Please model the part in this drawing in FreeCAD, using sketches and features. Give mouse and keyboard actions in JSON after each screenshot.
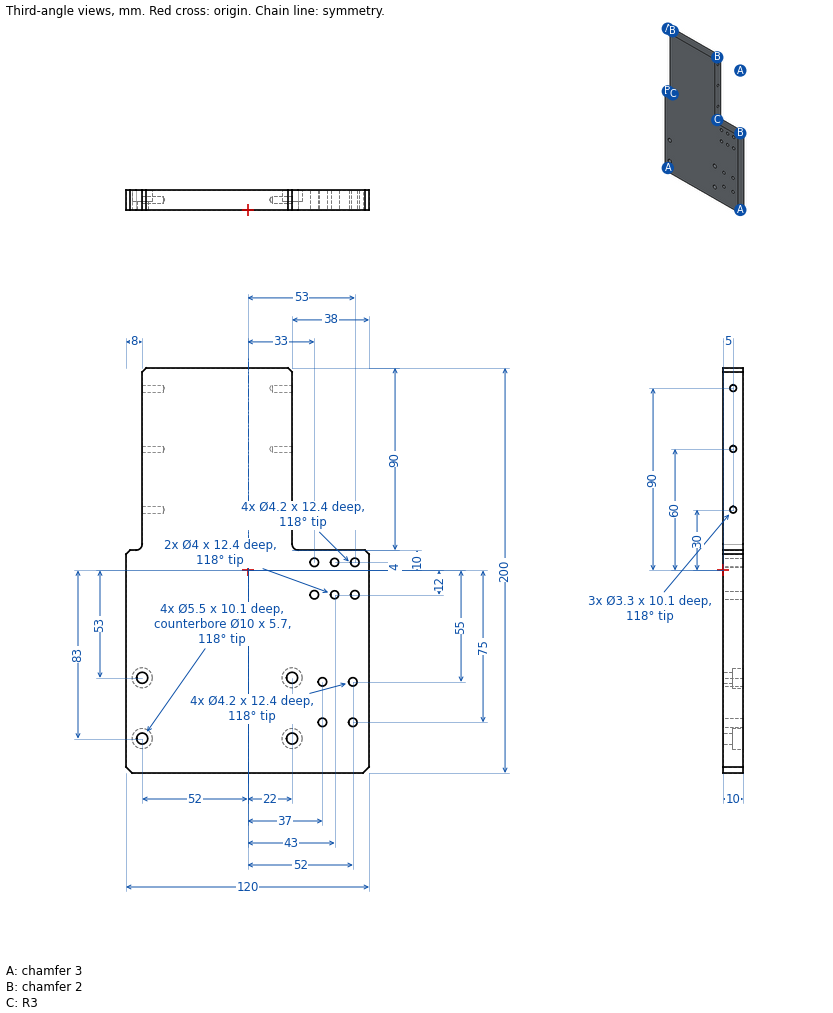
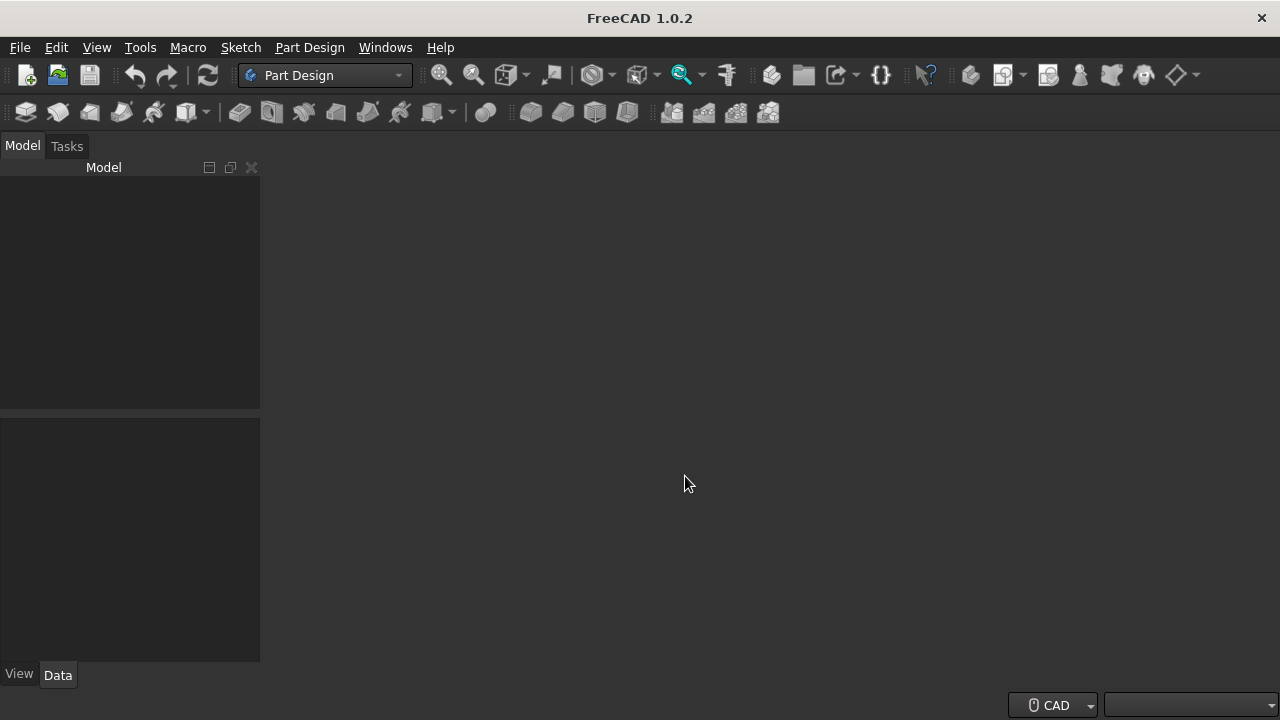
{"action": "left_click", "coordinate": [26, 76]}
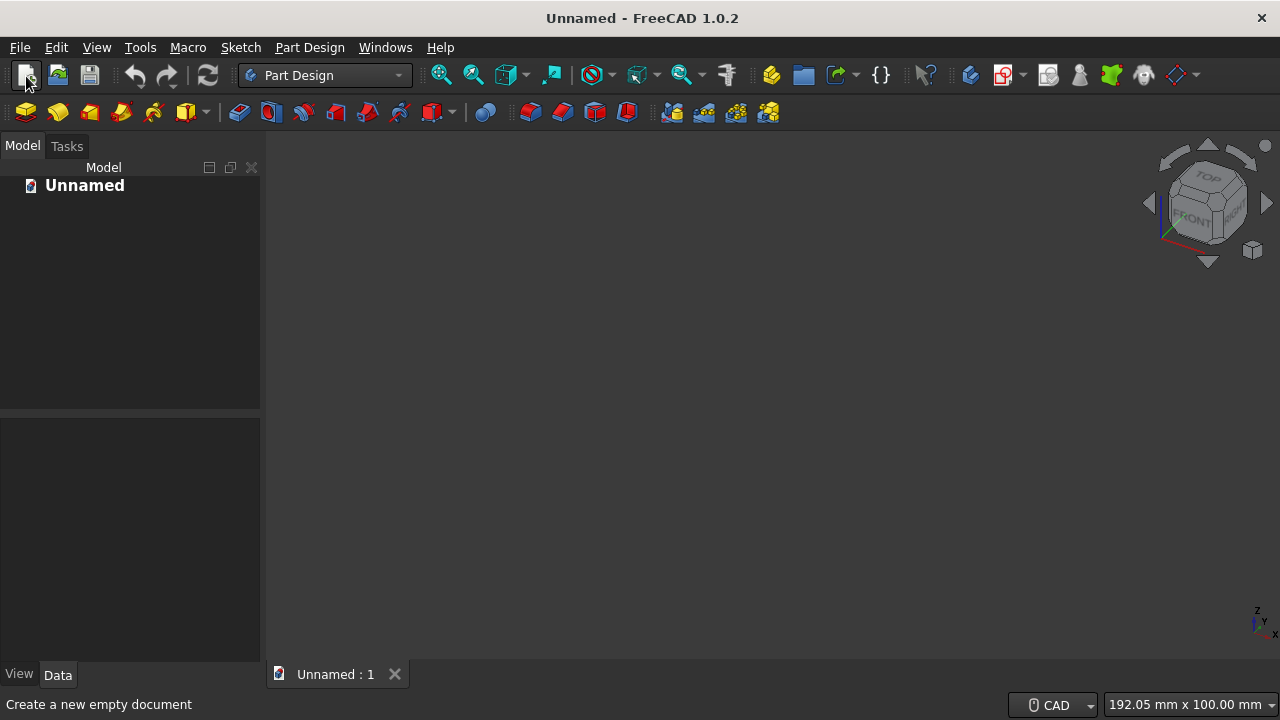
{"action": "left_click", "coordinate": [1004, 76]}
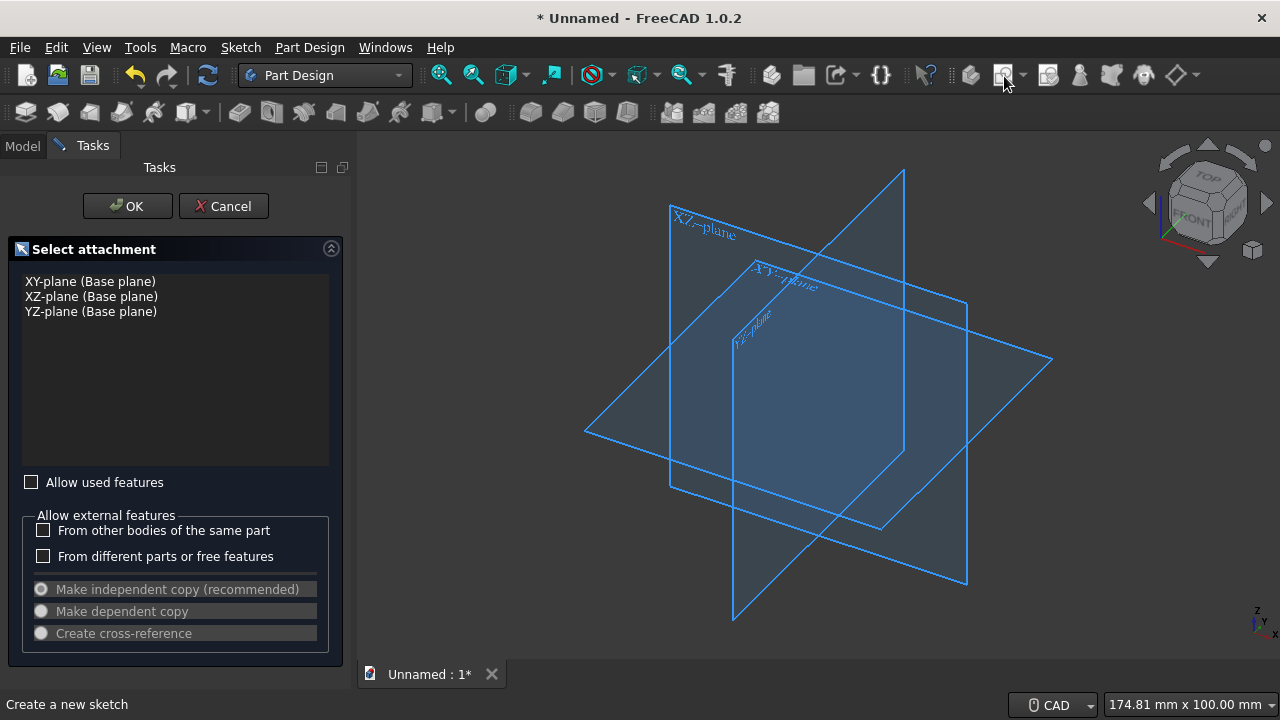
{"action": "left_click", "coordinate": [82, 296]}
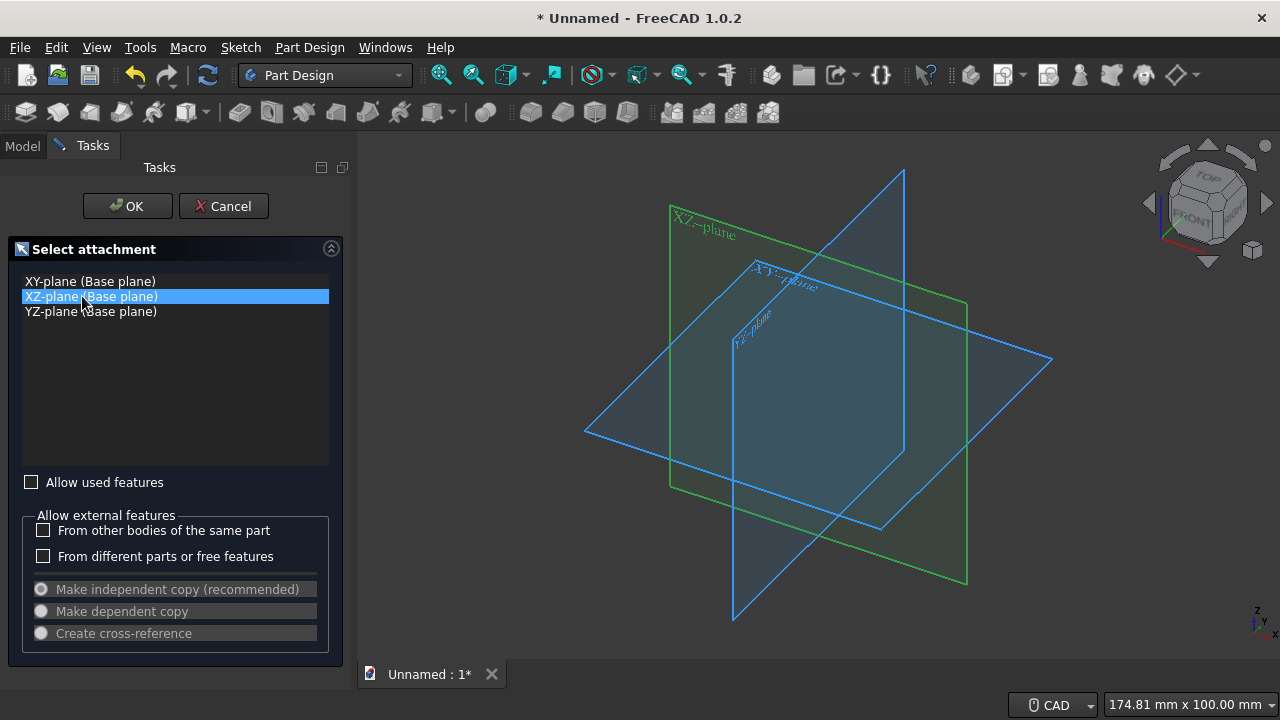
{"action": "left_click", "coordinate": [128, 206]}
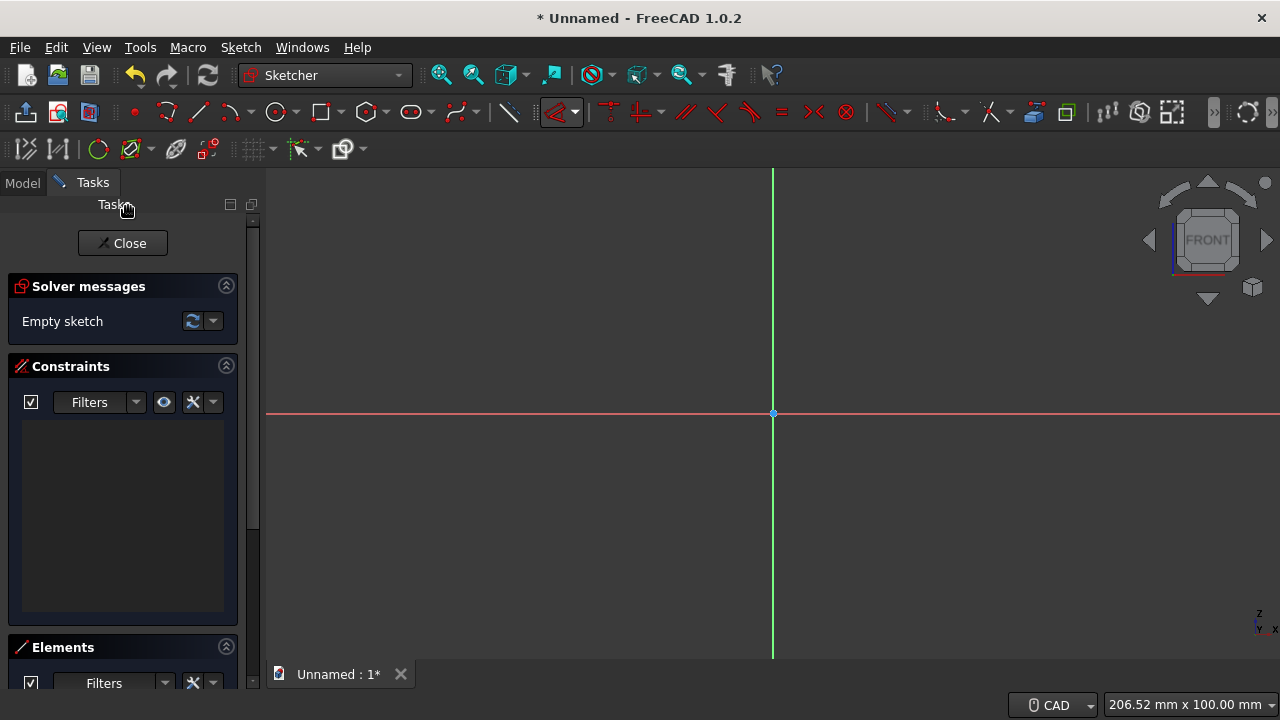
{"action": "scroll", "coordinate": [675, 413], "scroll_direction": "down", "scroll_amount": 6}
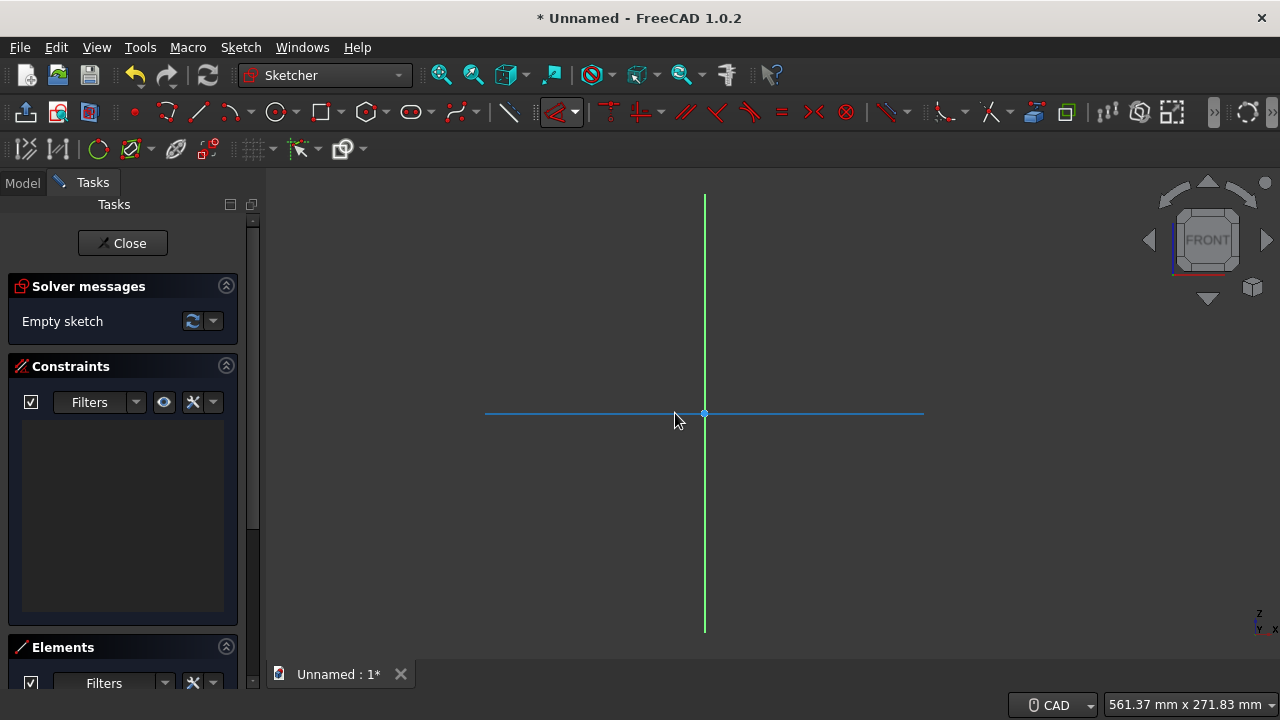
{"action": "key", "text": "g v"}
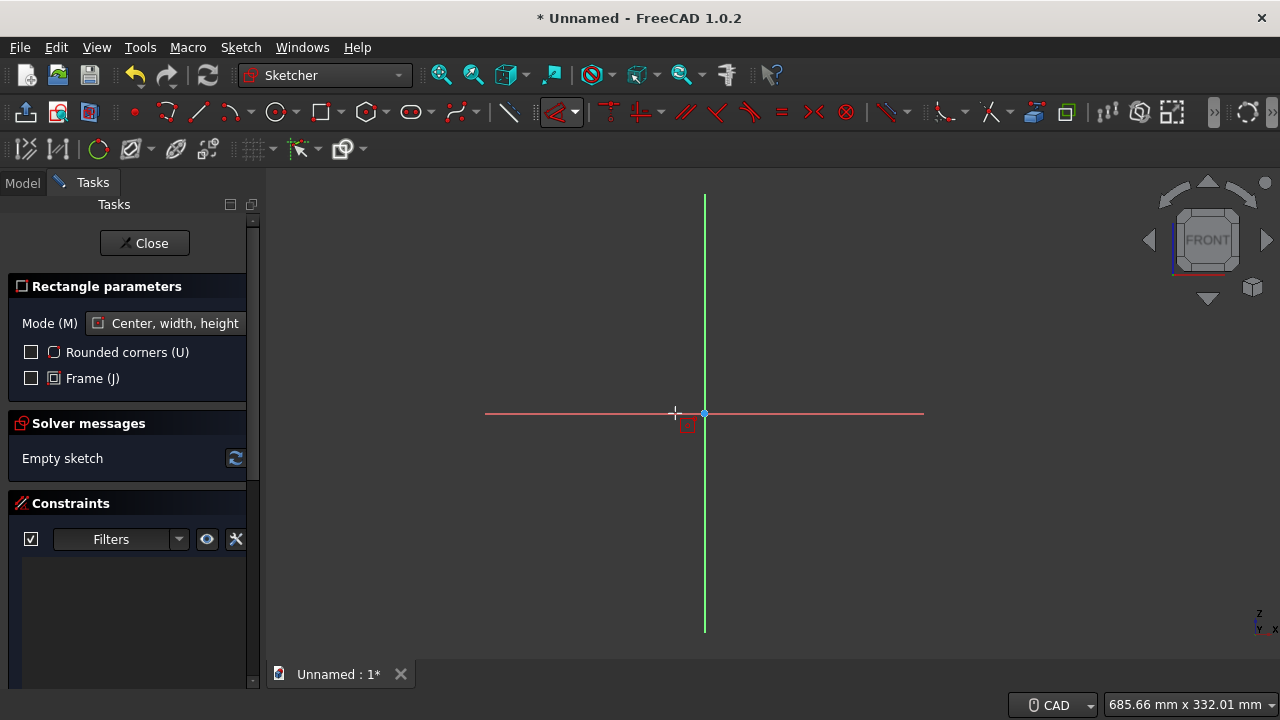
{"action": "left_click", "coordinate": [705, 414]}
{"action": "left_click", "coordinate": [794, 266]}
{"action": "key", "text": "Escape"}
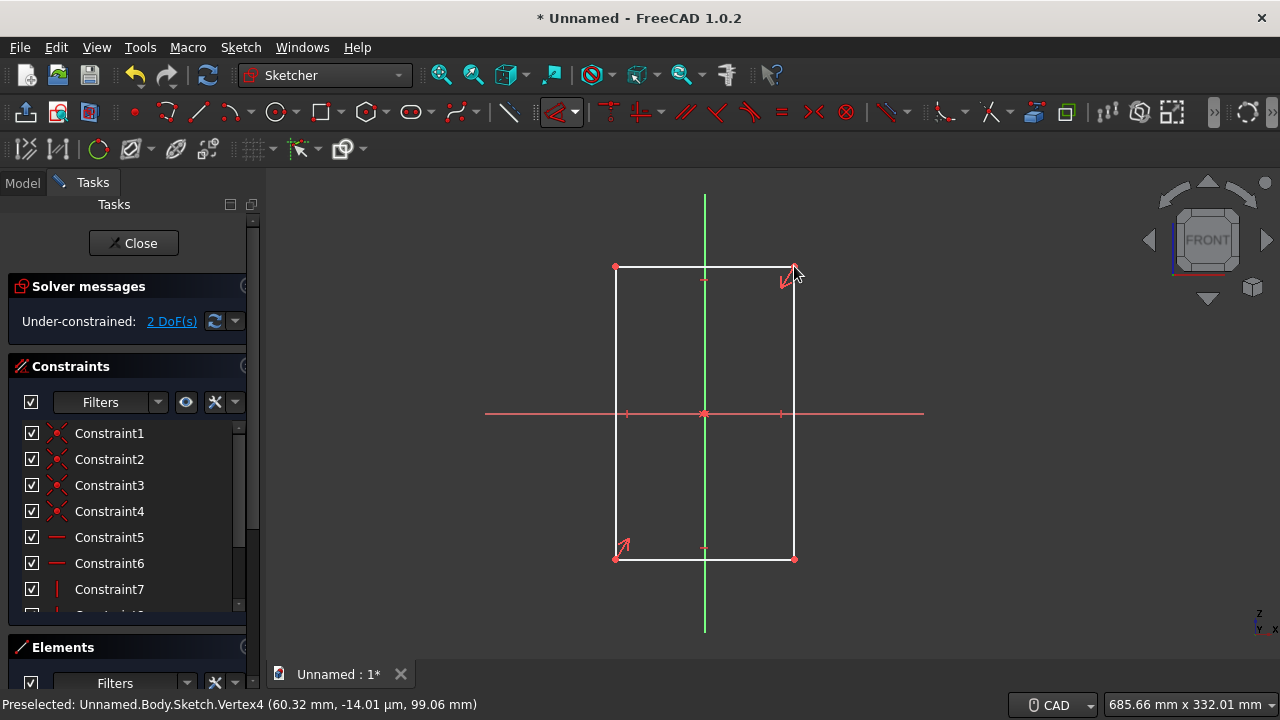
{"action": "left_click", "coordinate": [556, 112]}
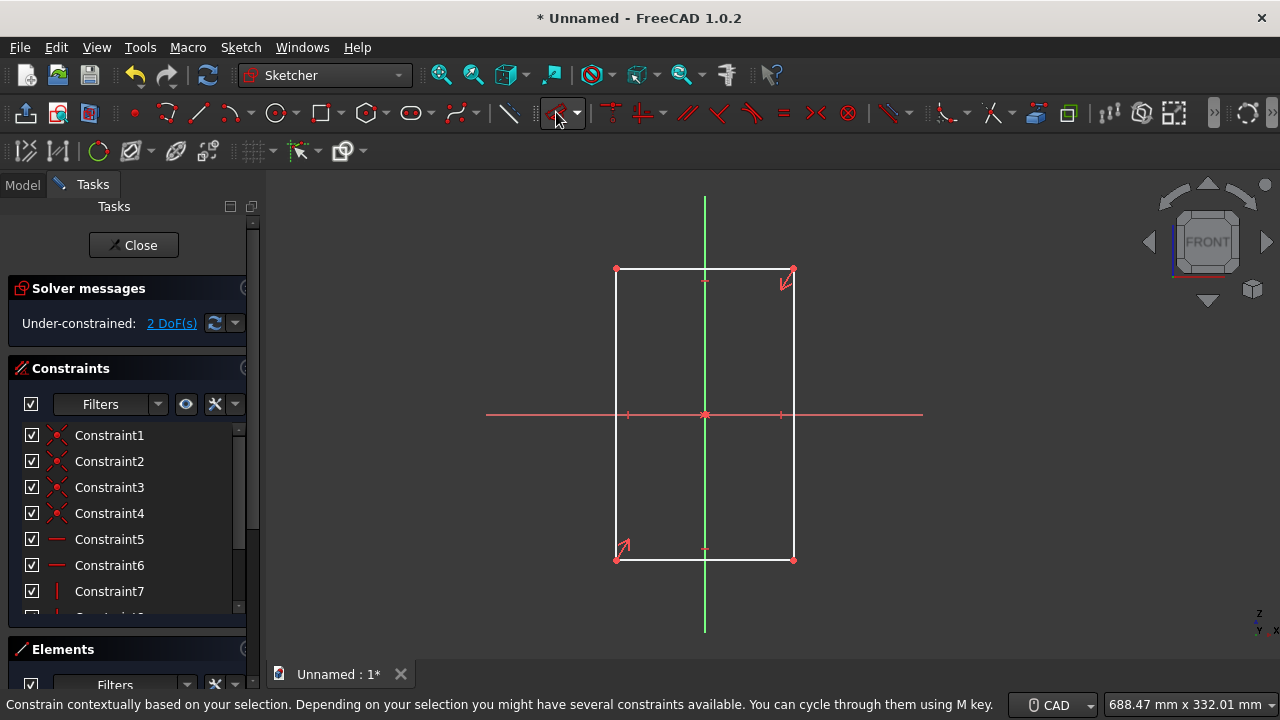
{"action": "left_click", "coordinate": [670, 560]}
{"action": "left_click", "coordinate": [664, 594]}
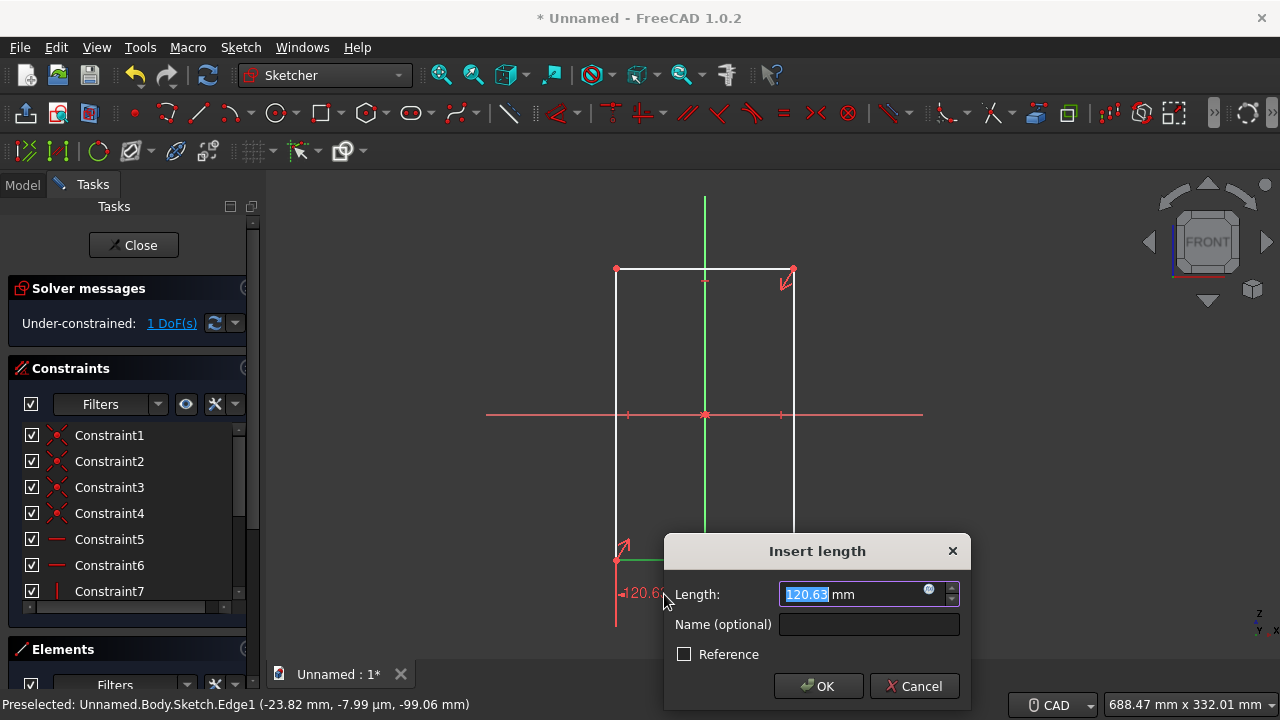
{"action": "type", "text": "120"}
{"action": "key", "text": "Return"}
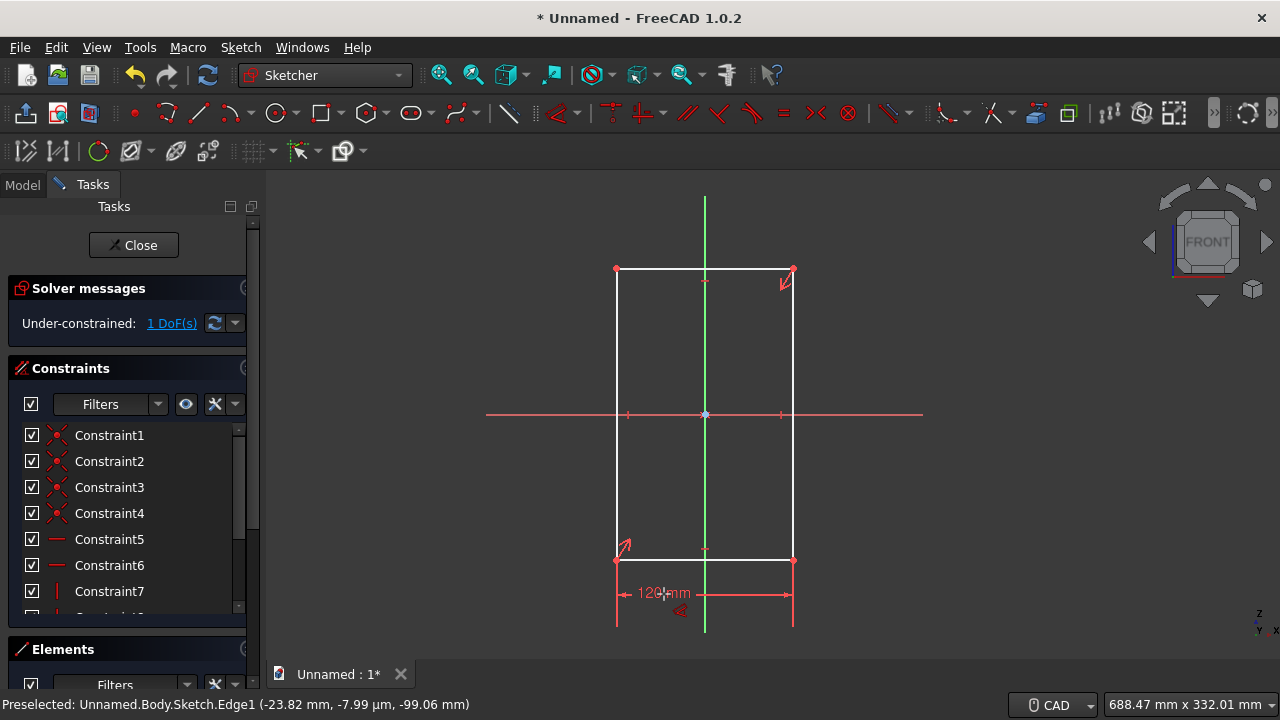
{"action": "left_click", "coordinate": [793, 473]}
{"action": "left_click", "coordinate": [827, 347]}